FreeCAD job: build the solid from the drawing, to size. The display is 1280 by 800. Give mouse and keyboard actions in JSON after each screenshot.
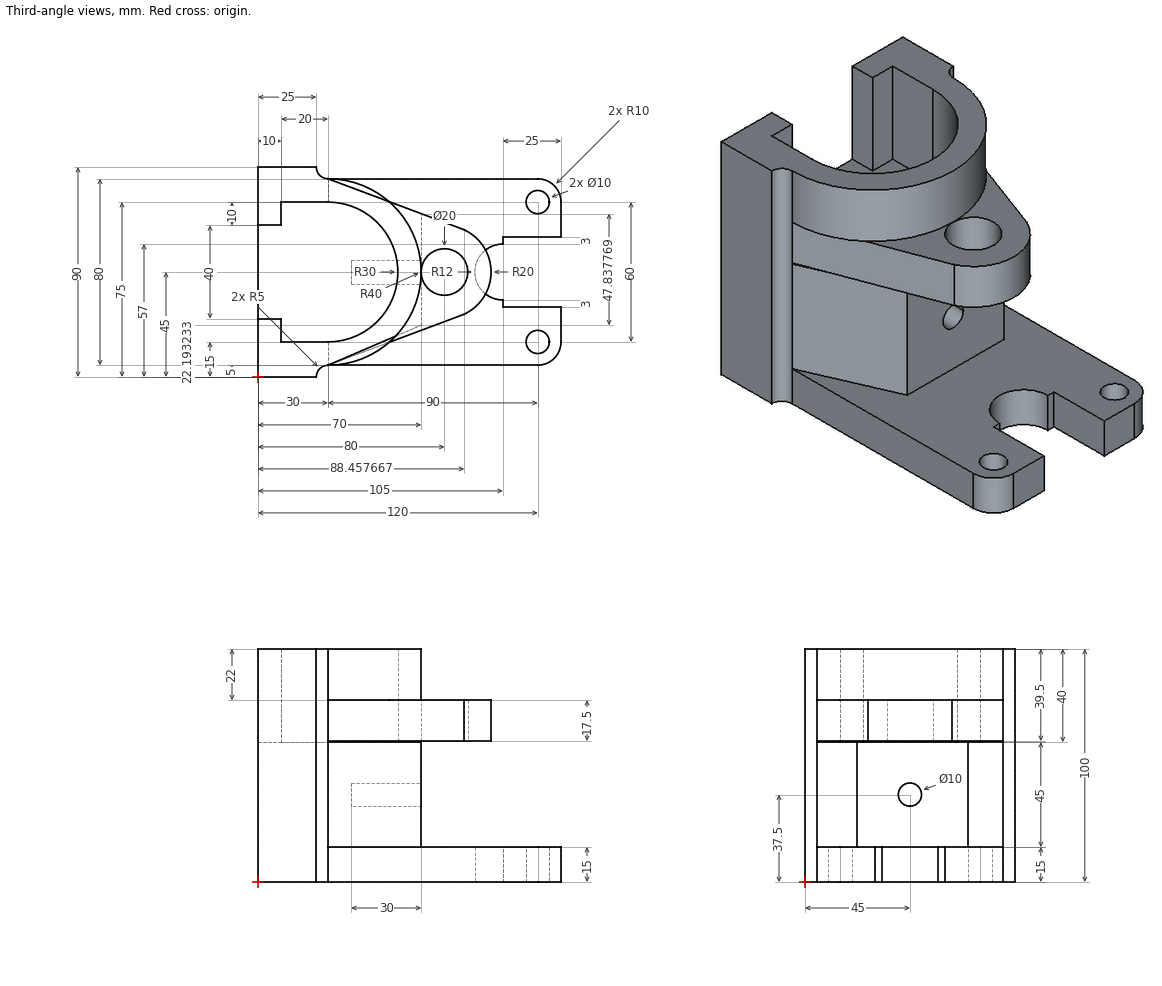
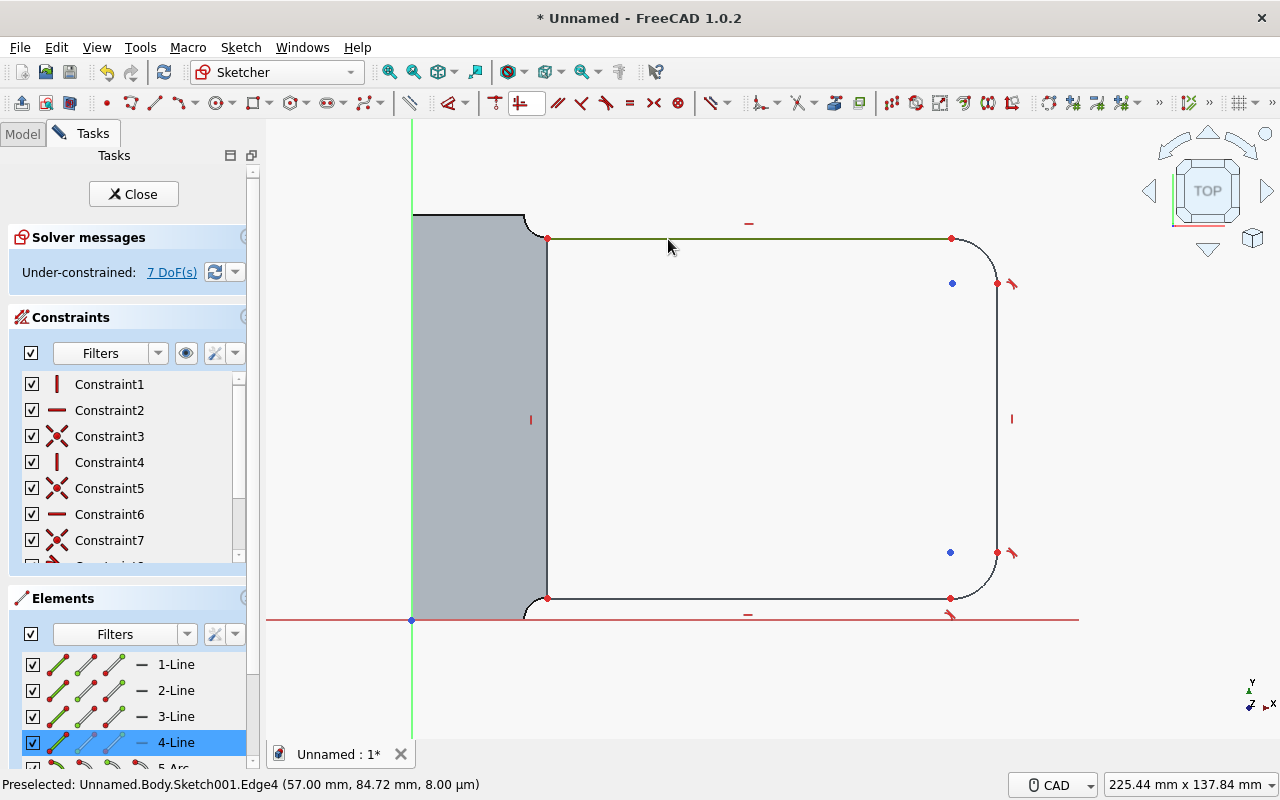
{"action": "left_click", "coordinate": [992, 263]}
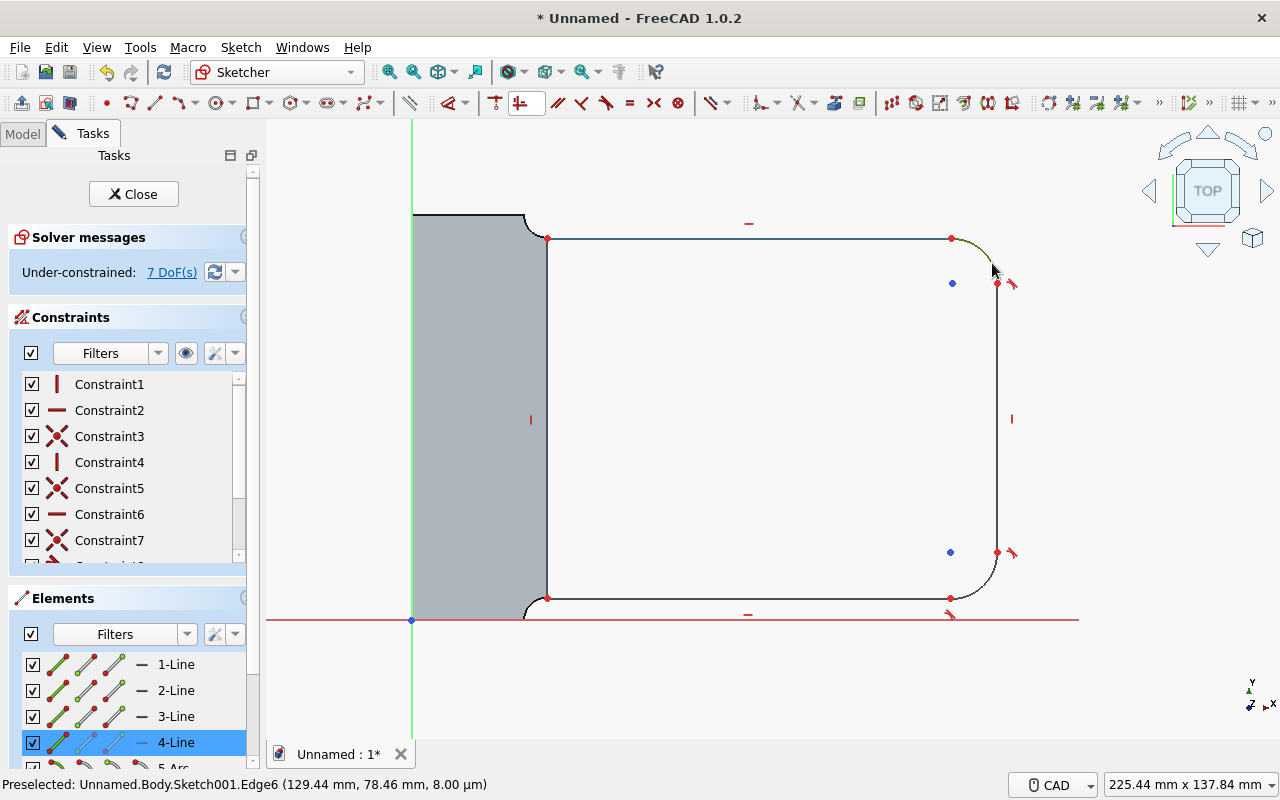
{"action": "key", "text": "t"}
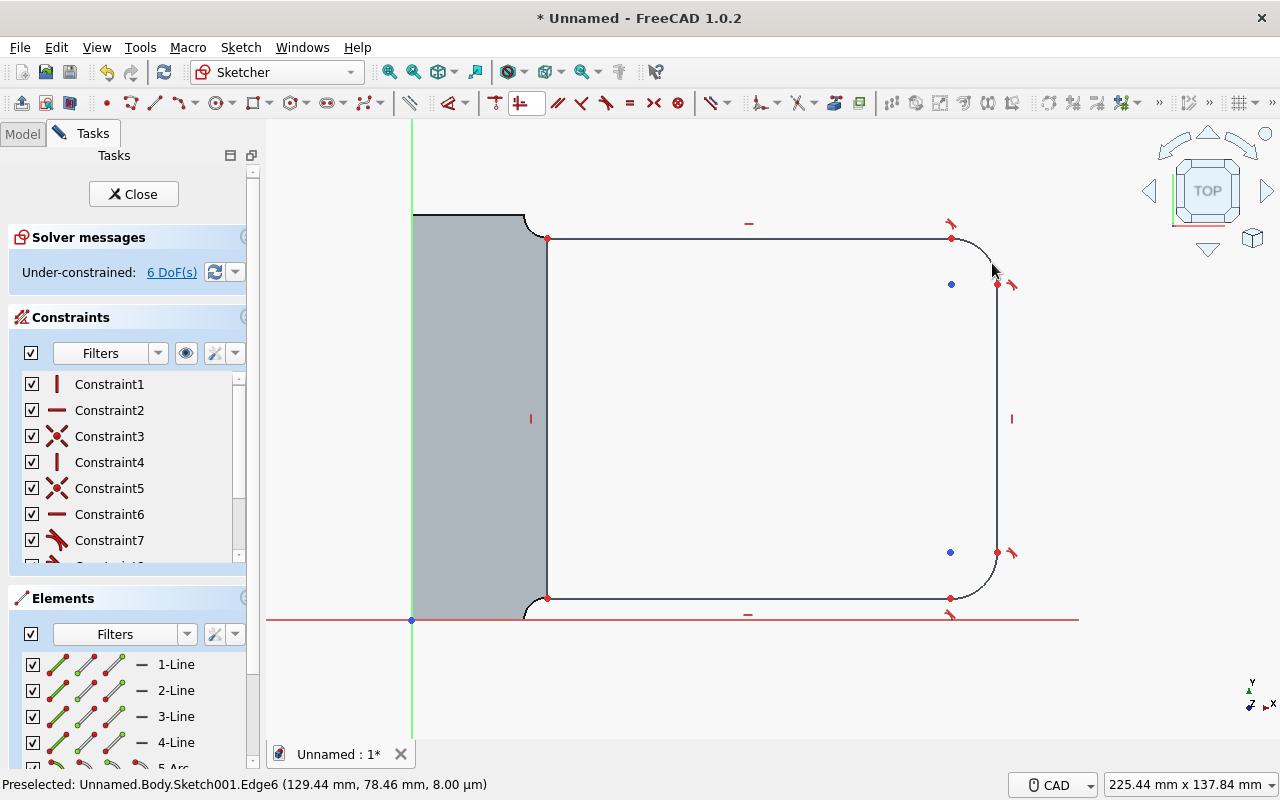
{"action": "left_click", "coordinate": [972, 594]}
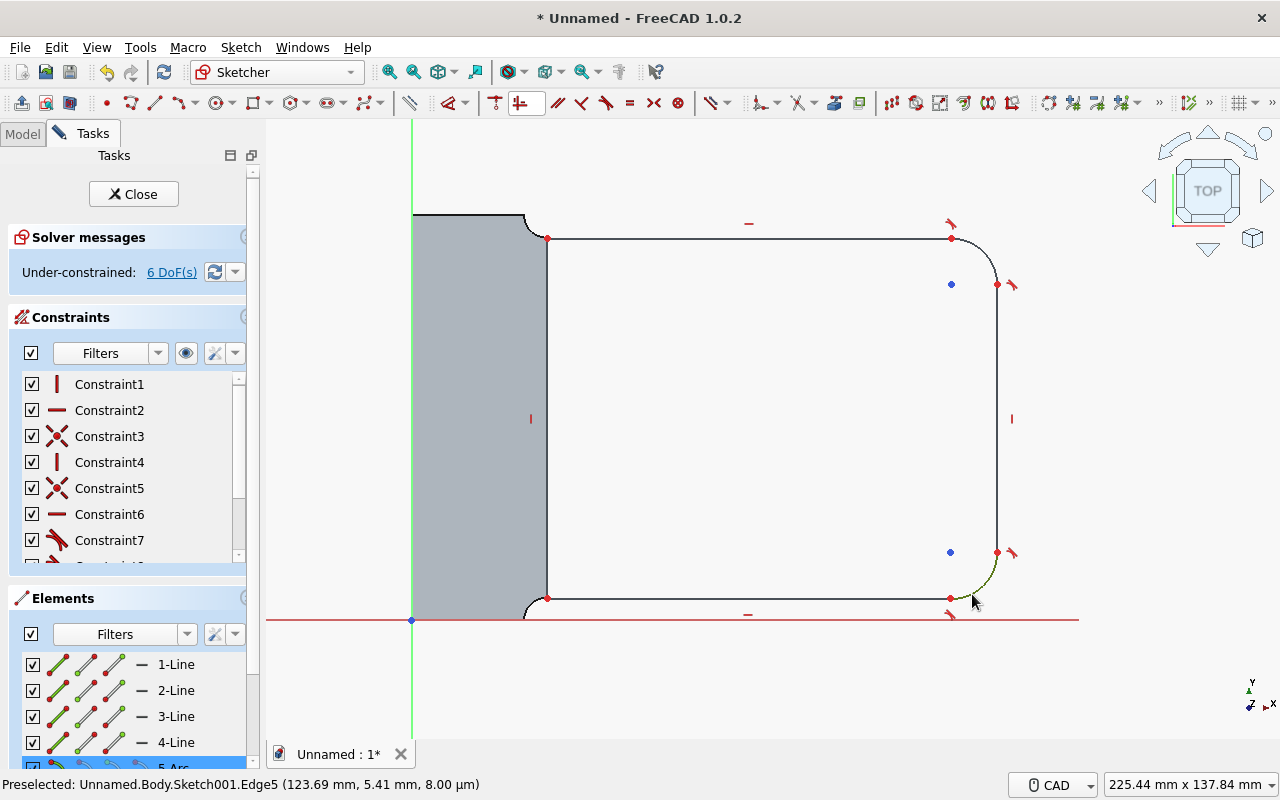
{"action": "left_click", "coordinate": [992, 264]}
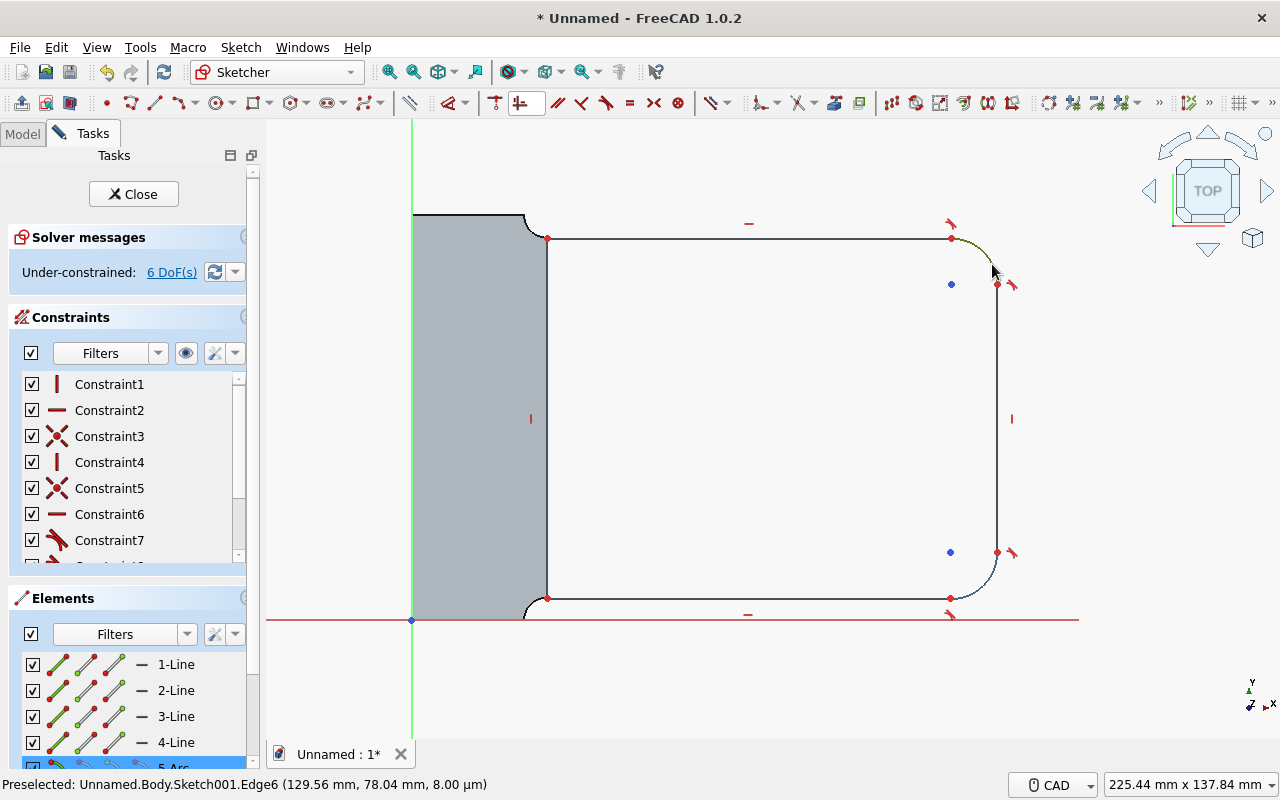
{"action": "key", "text": "e"}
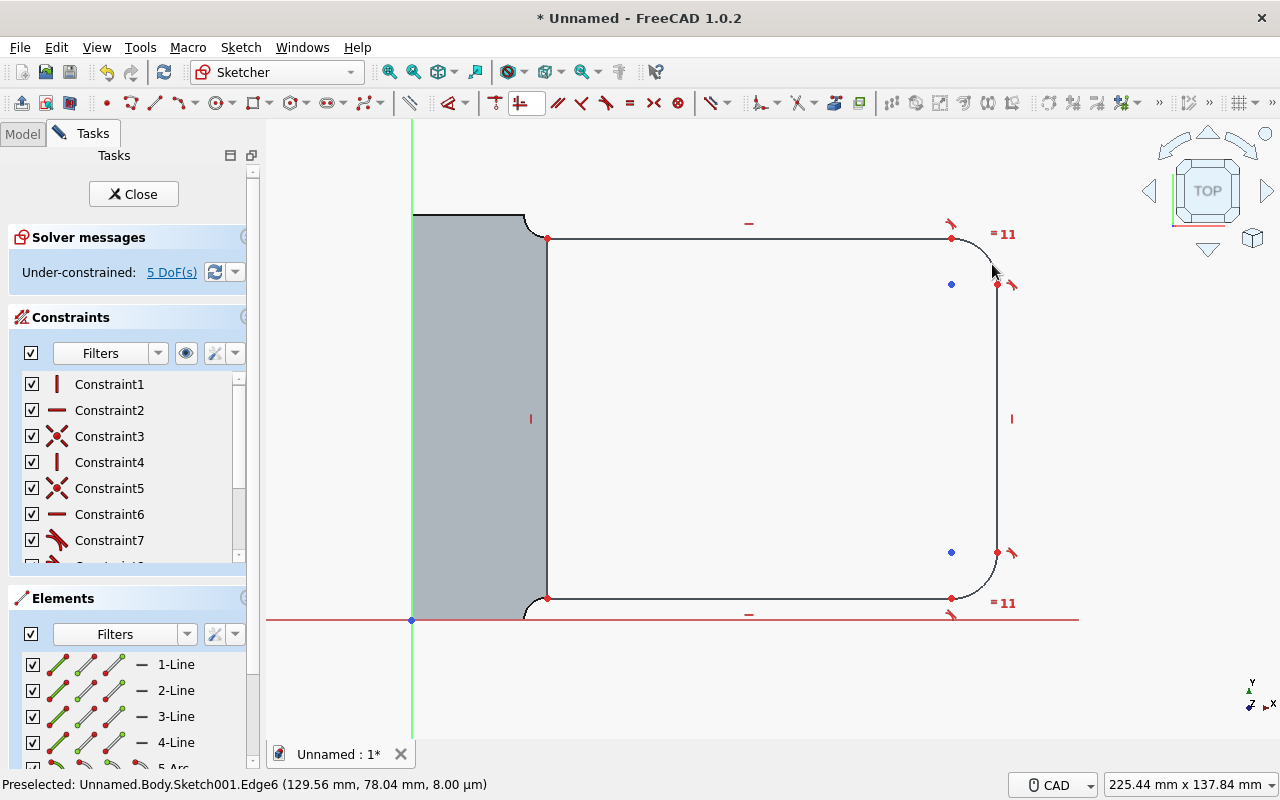
{"action": "left_click", "coordinate": [448, 104]}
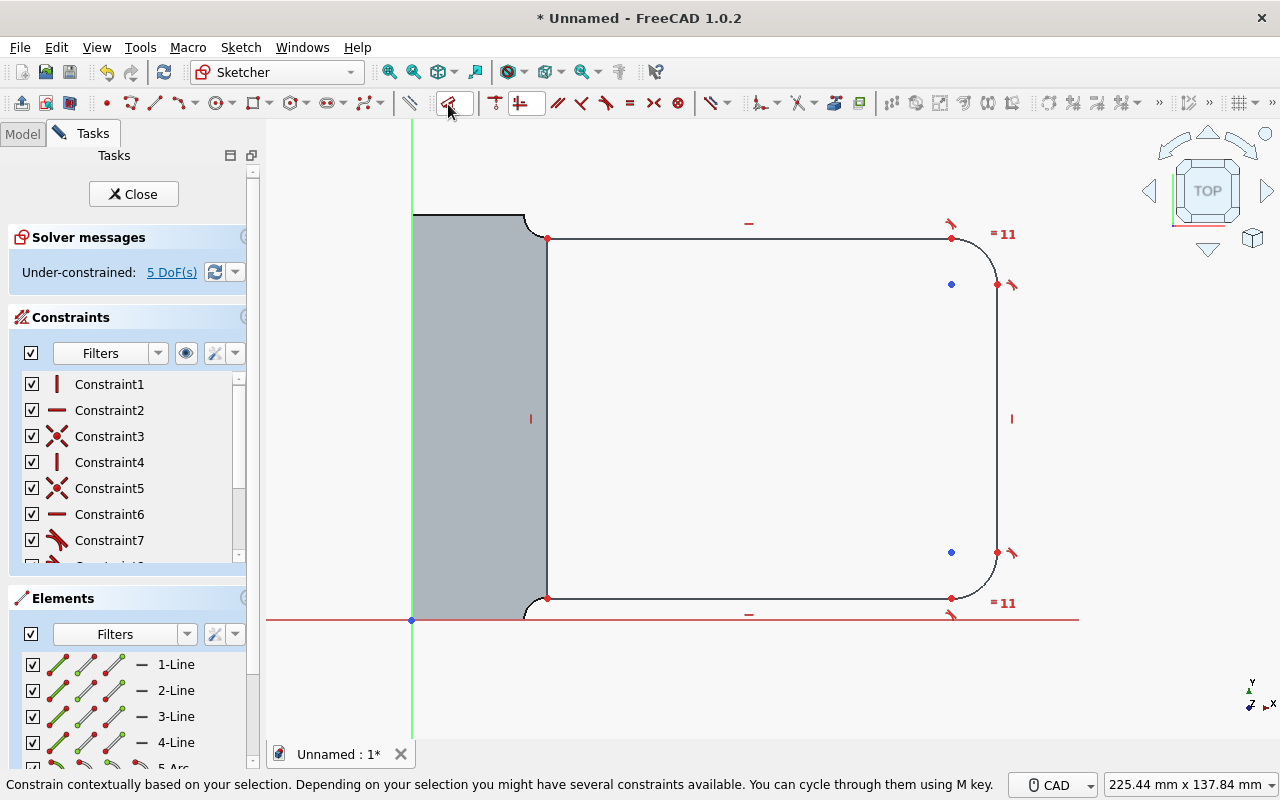
{"action": "left_click", "coordinate": [972, 594]}
{"action": "left_click", "coordinate": [1016, 597]}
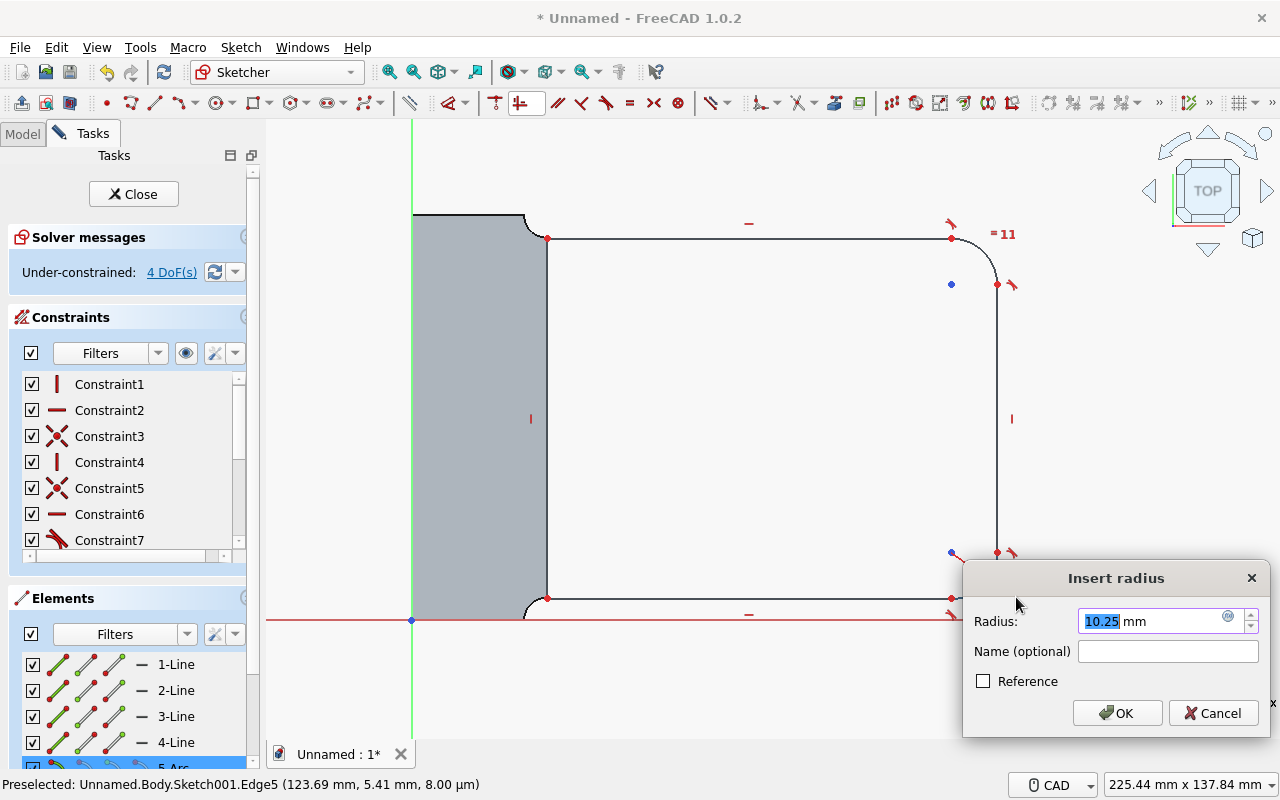
{"action": "type", "text": "10"}
{"action": "key", "text": "Return"}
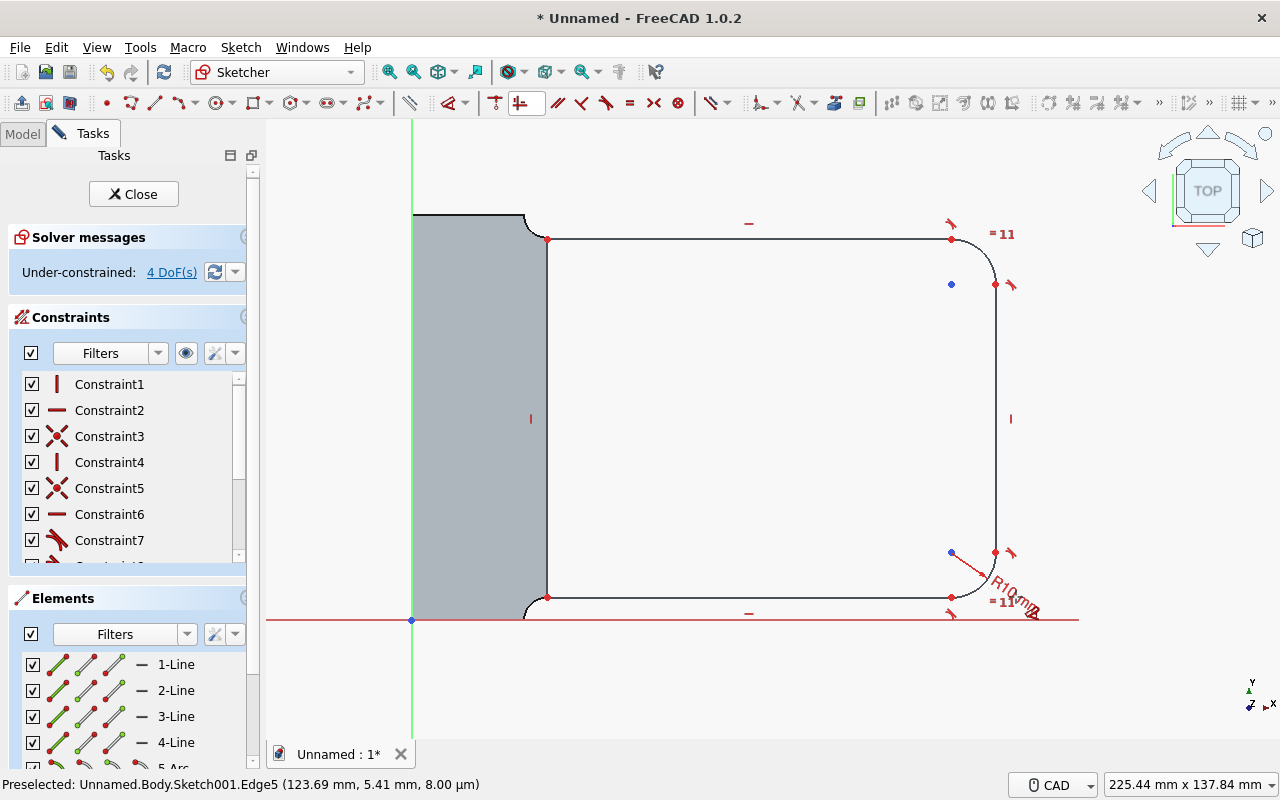
{"action": "left_click", "coordinate": [996, 365]}
{"action": "left_click", "coordinate": [1030, 419]}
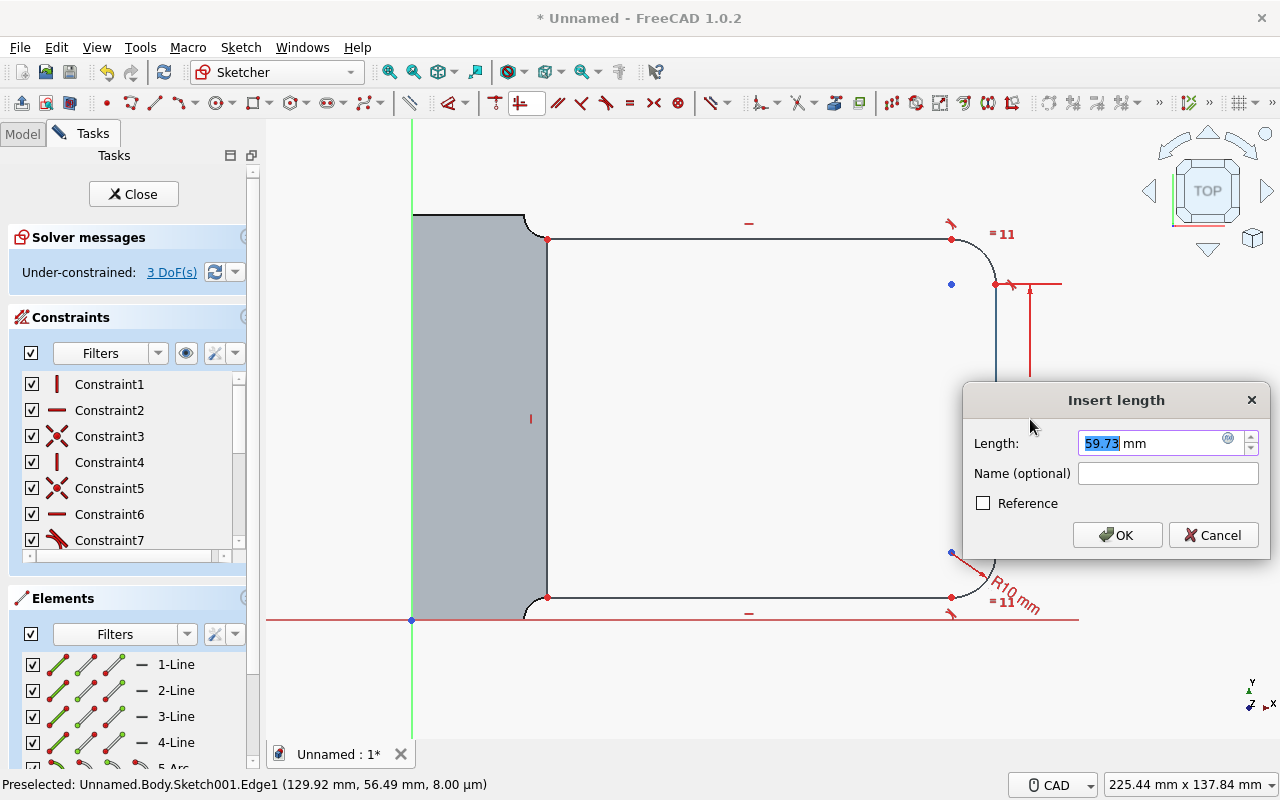
{"action": "type", "text": "60"}
{"action": "key", "text": "Return"}